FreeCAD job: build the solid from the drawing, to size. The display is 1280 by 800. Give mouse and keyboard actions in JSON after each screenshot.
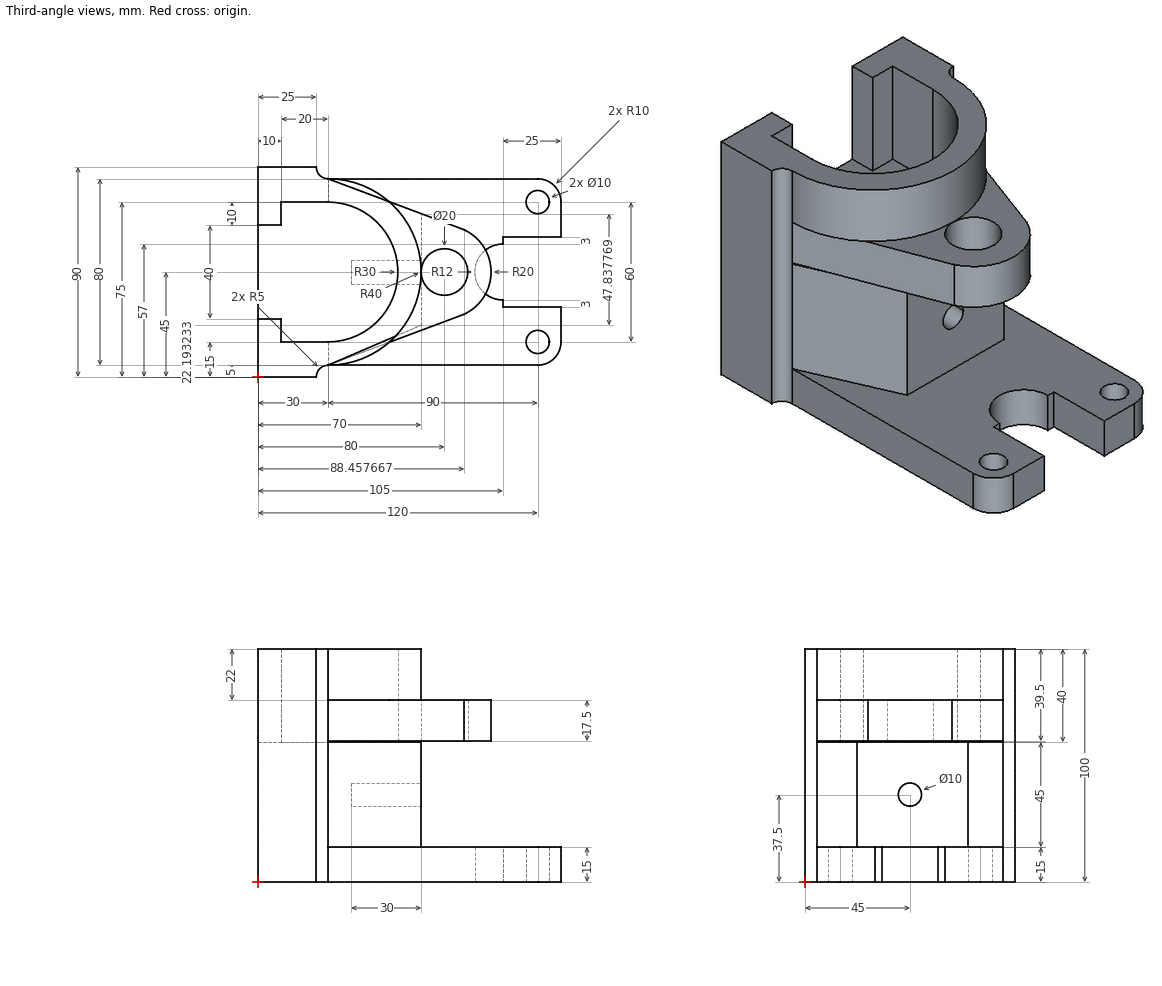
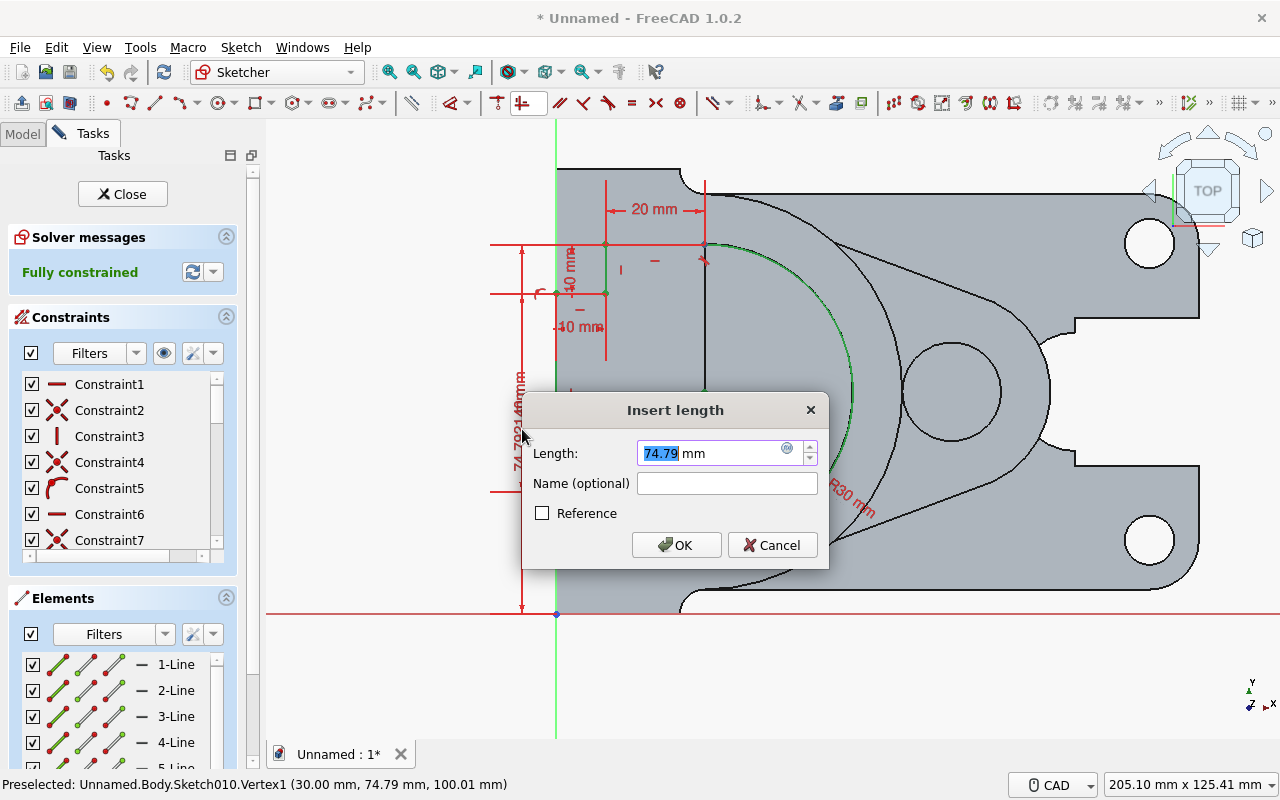
{"action": "type", "text": "75"}
{"action": "key", "text": "Return"}
{"action": "key", "text": "Escape"}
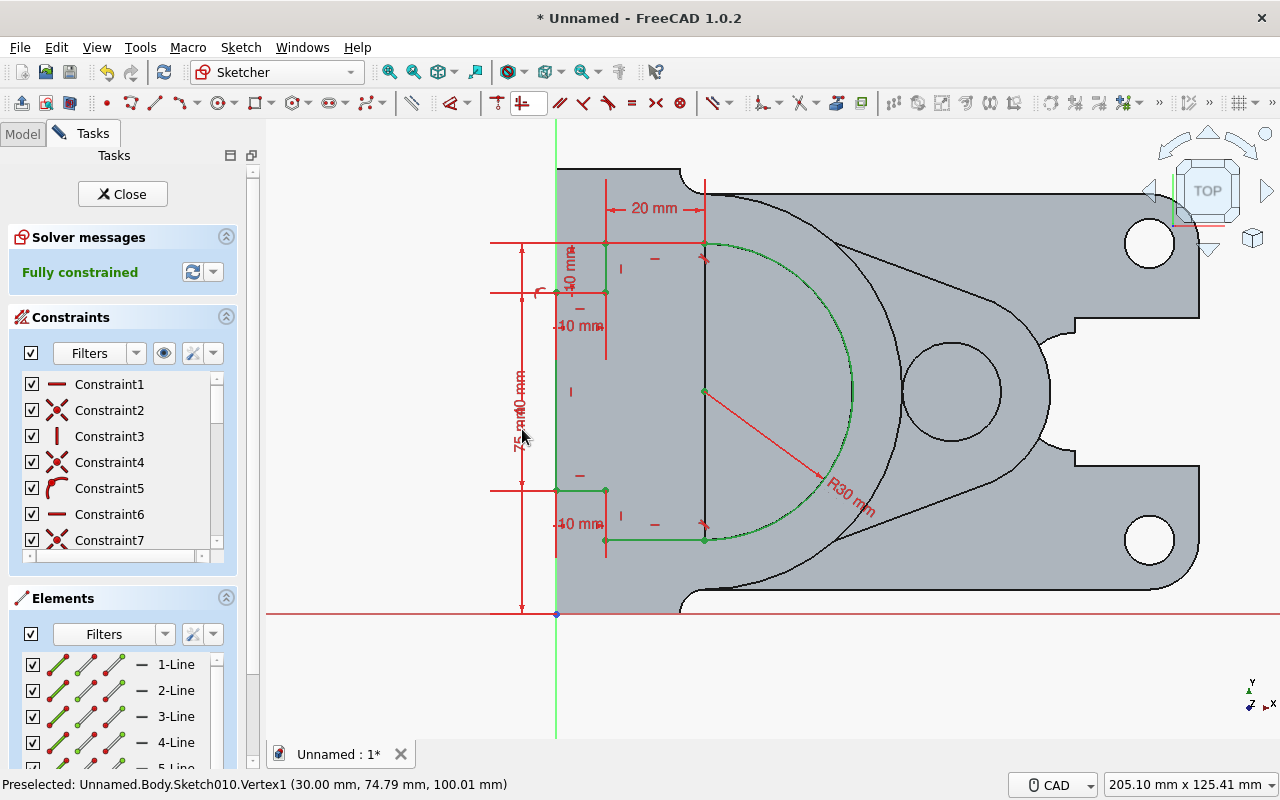
{"action": "left_click", "coordinate": [123, 194]}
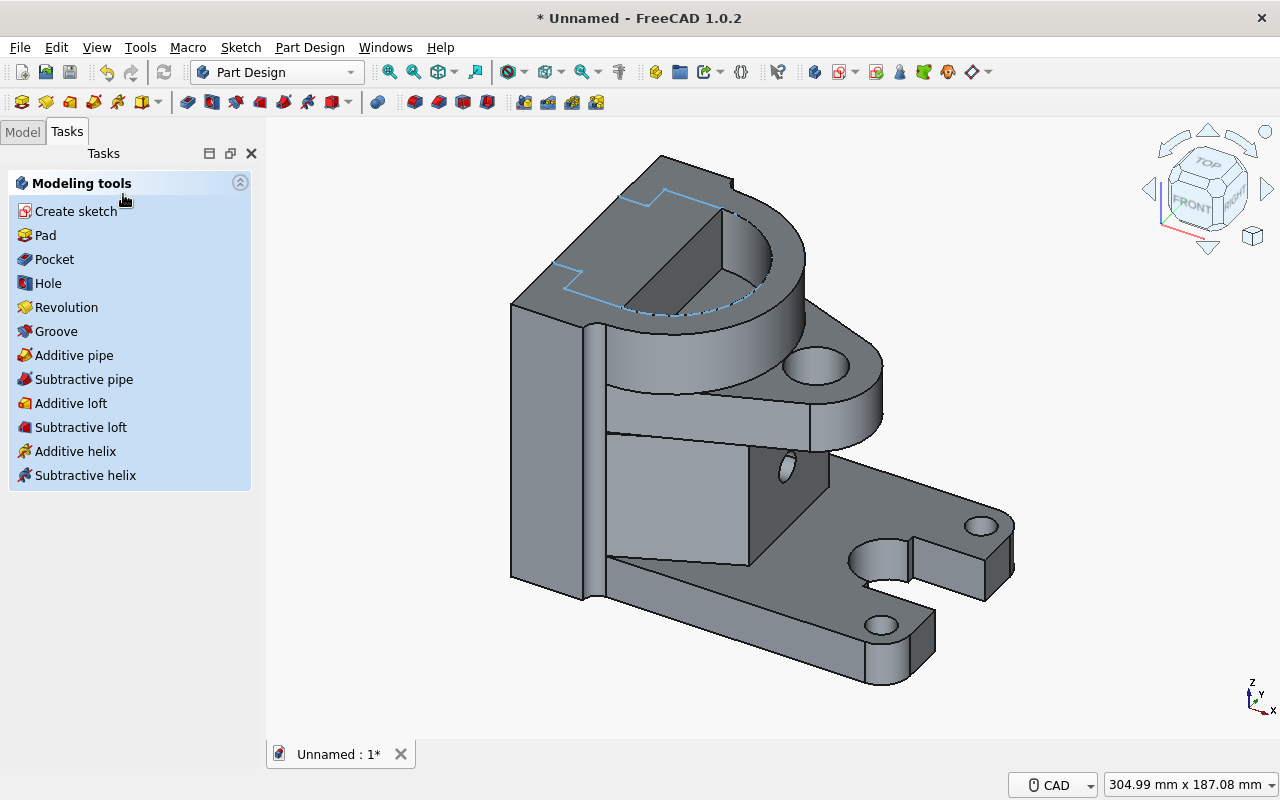
{"action": "left_click", "coordinate": [188, 102]}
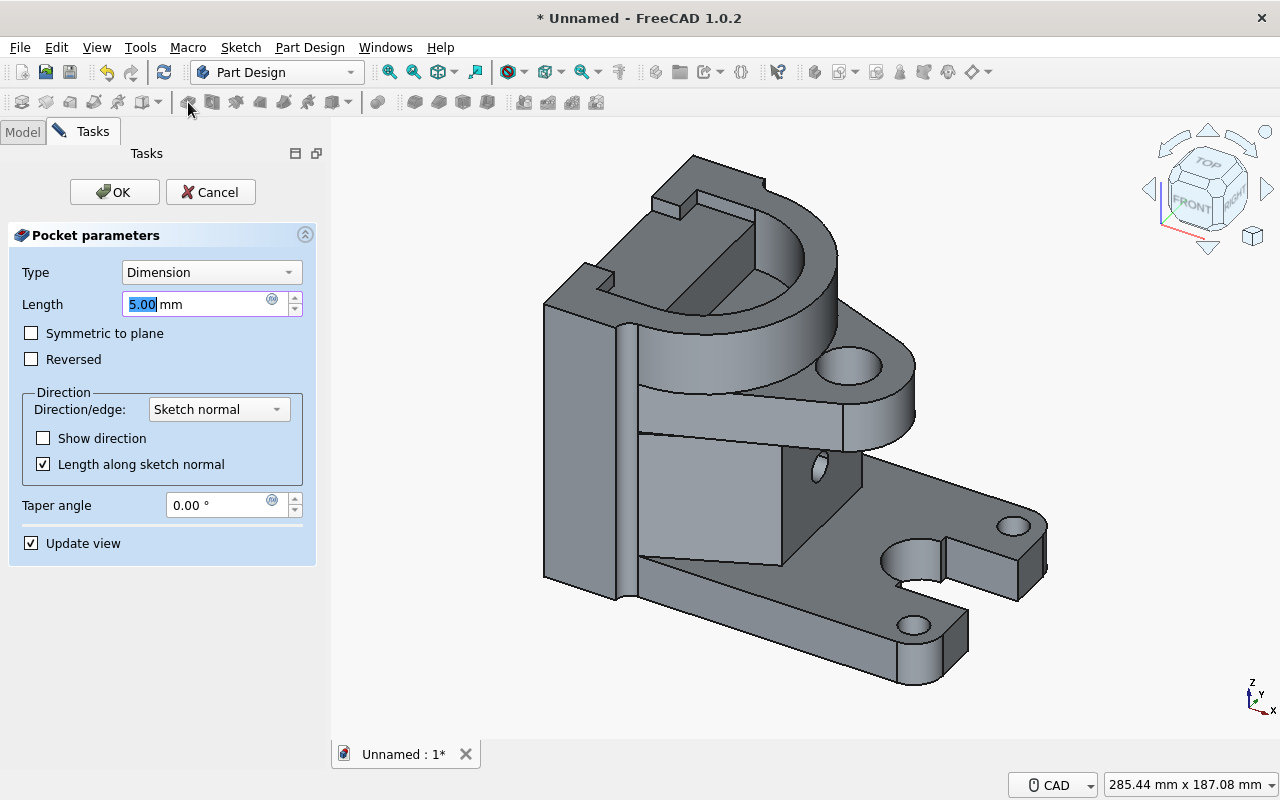
{"action": "type", "text": "40"}
{"action": "key", "text": "Tab"}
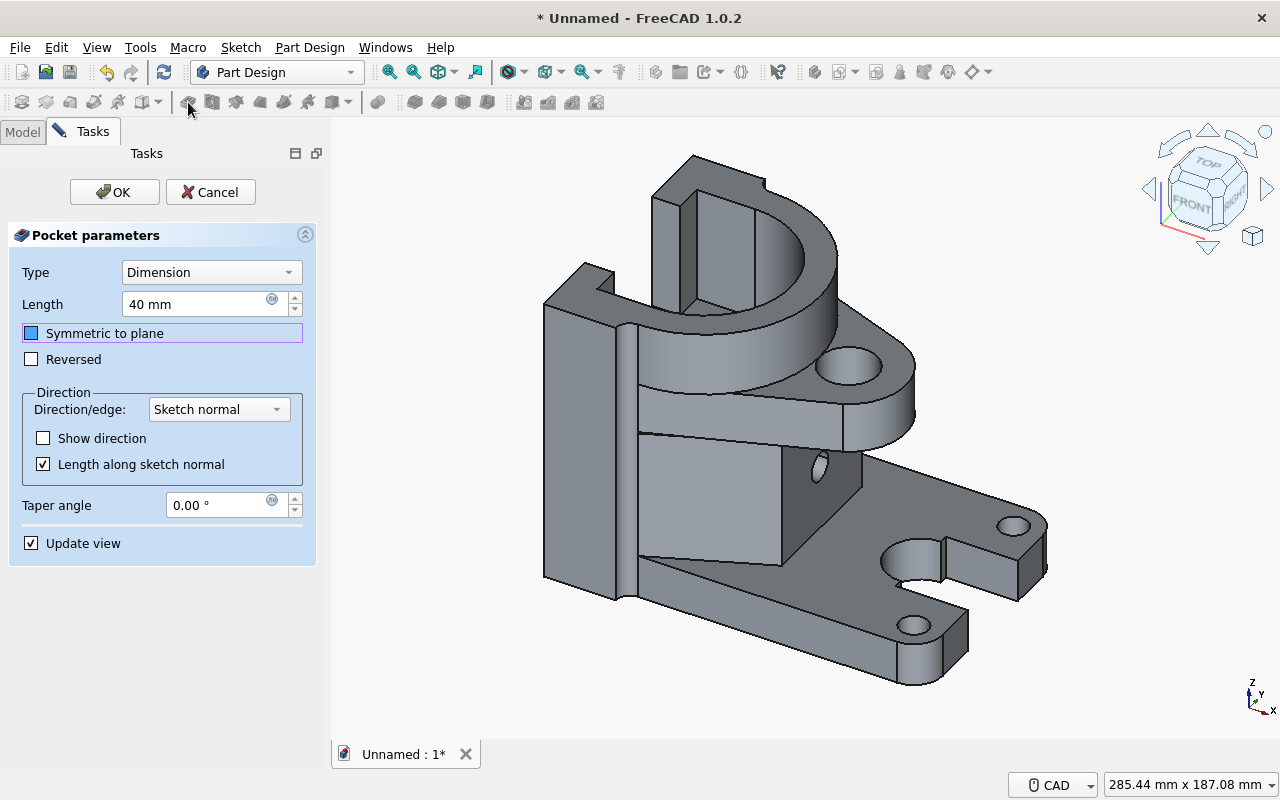
{"action": "left_click", "coordinate": [115, 192]}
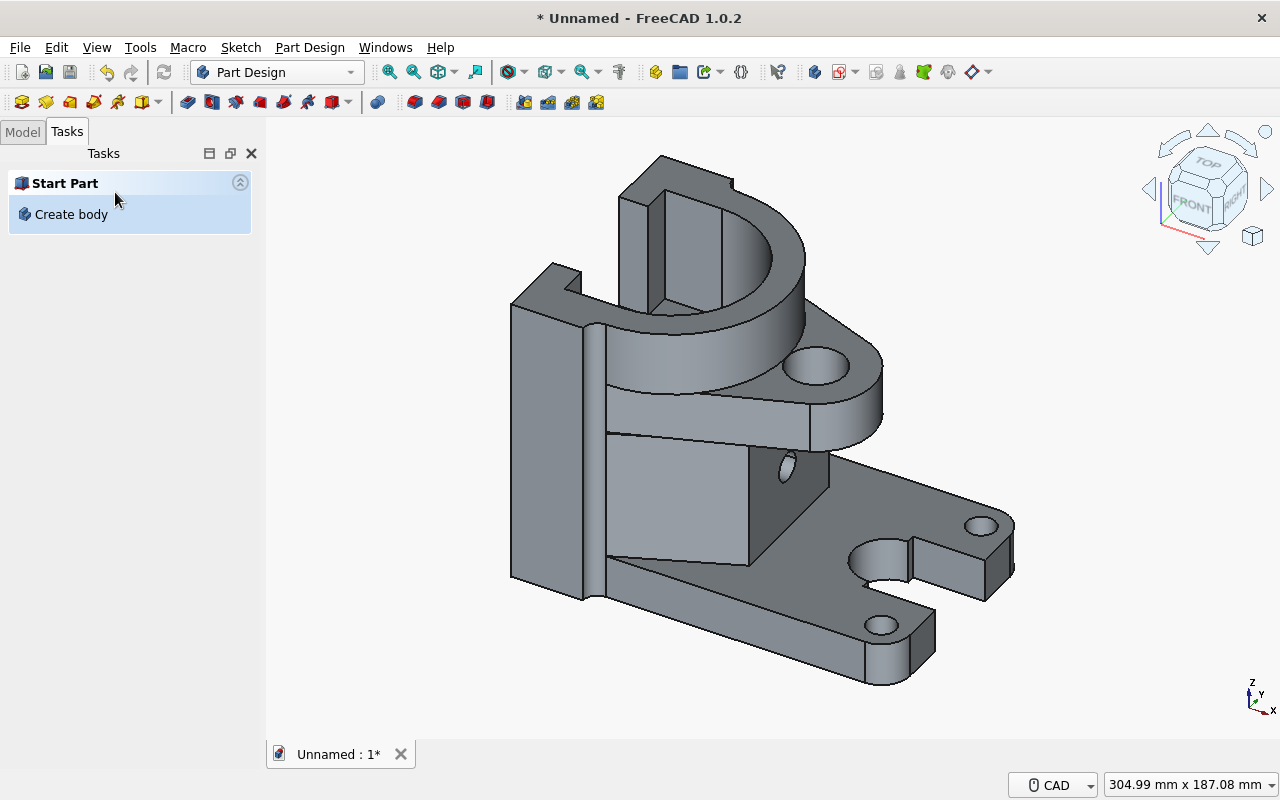
{"action": "key", "text": "0"}